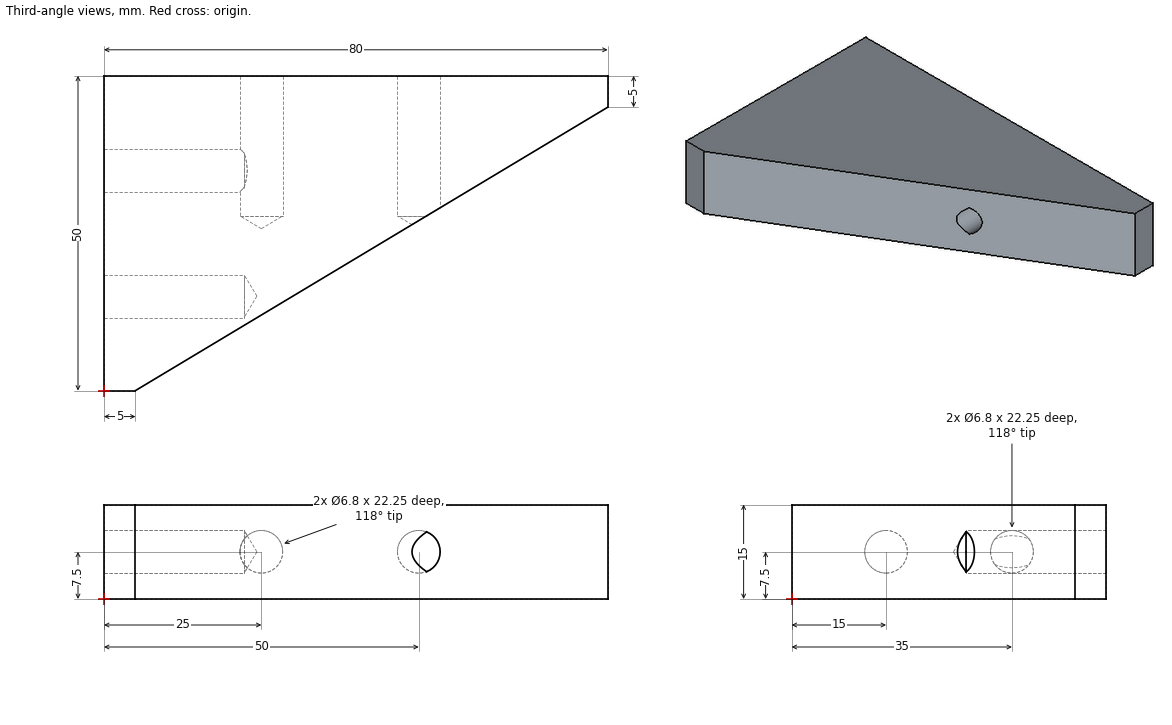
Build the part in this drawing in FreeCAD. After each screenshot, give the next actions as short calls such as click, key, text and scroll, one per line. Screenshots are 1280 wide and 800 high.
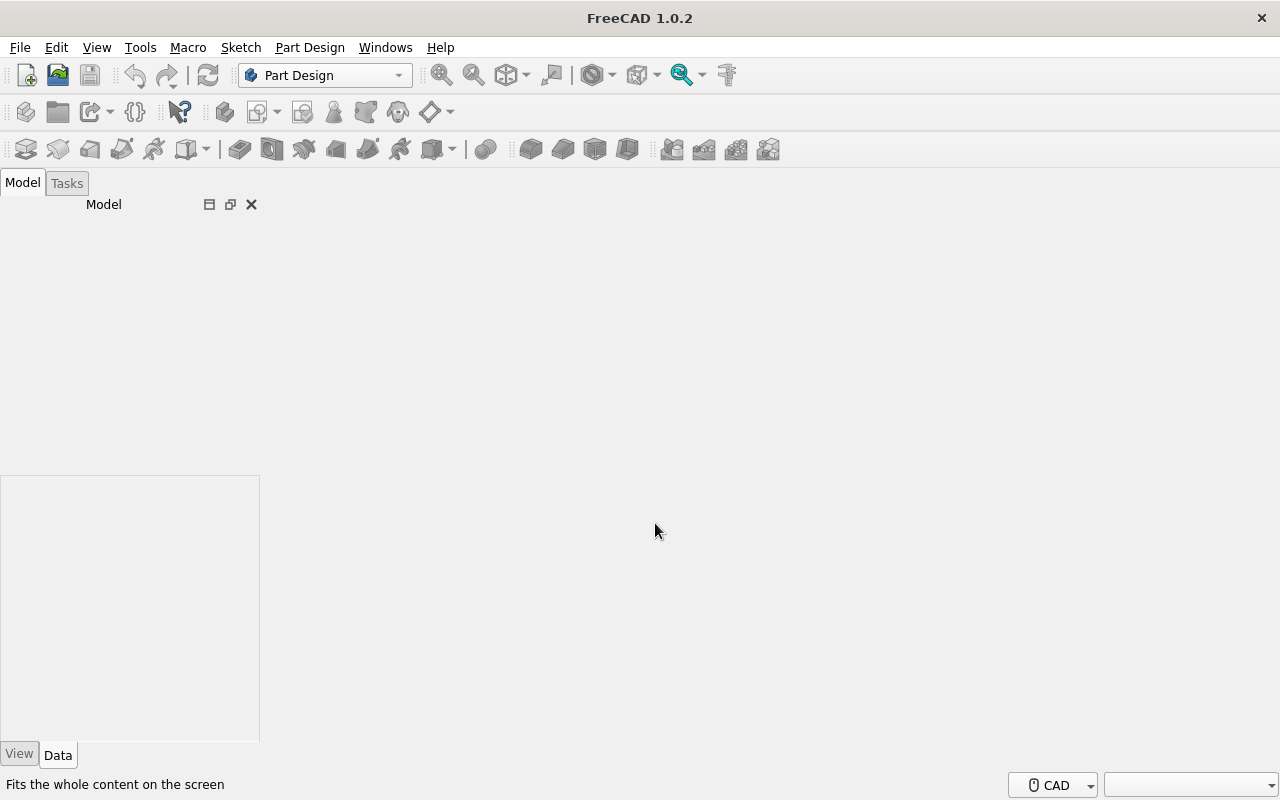
click(26, 76)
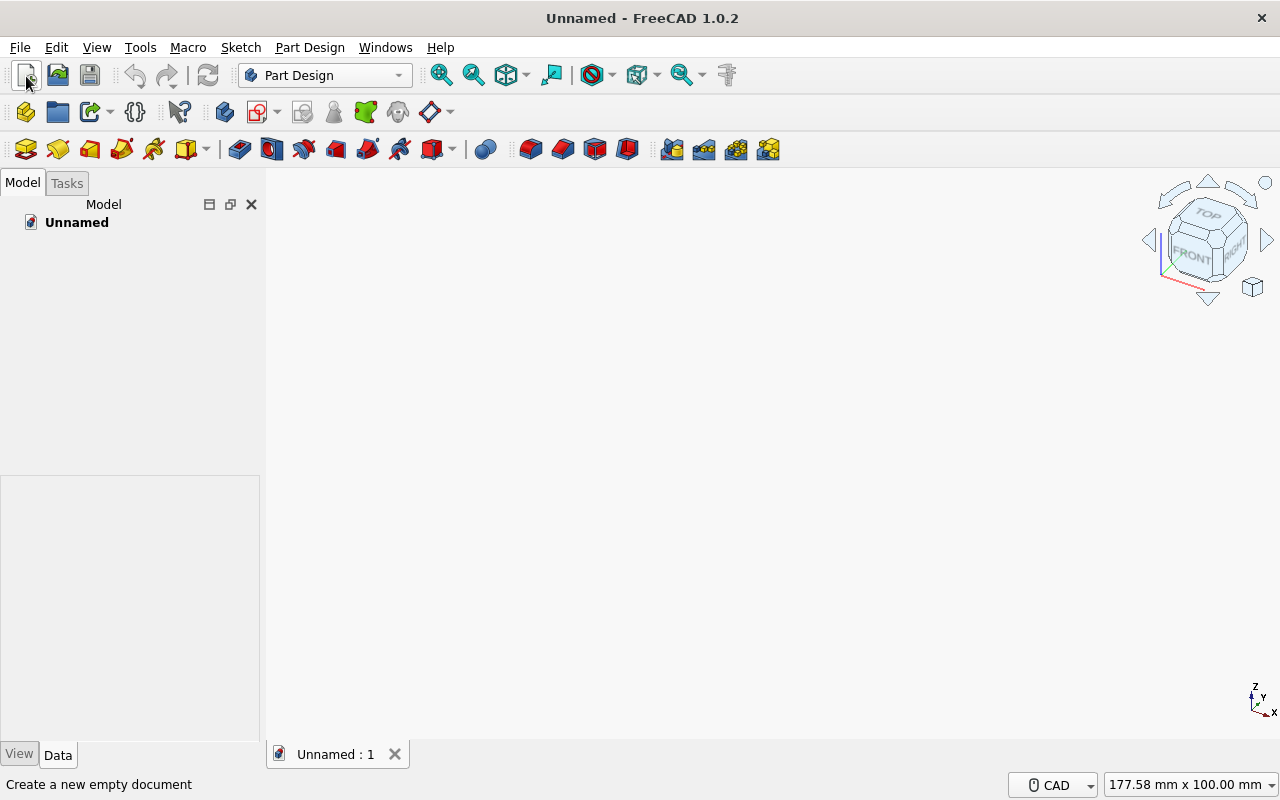
click(258, 112)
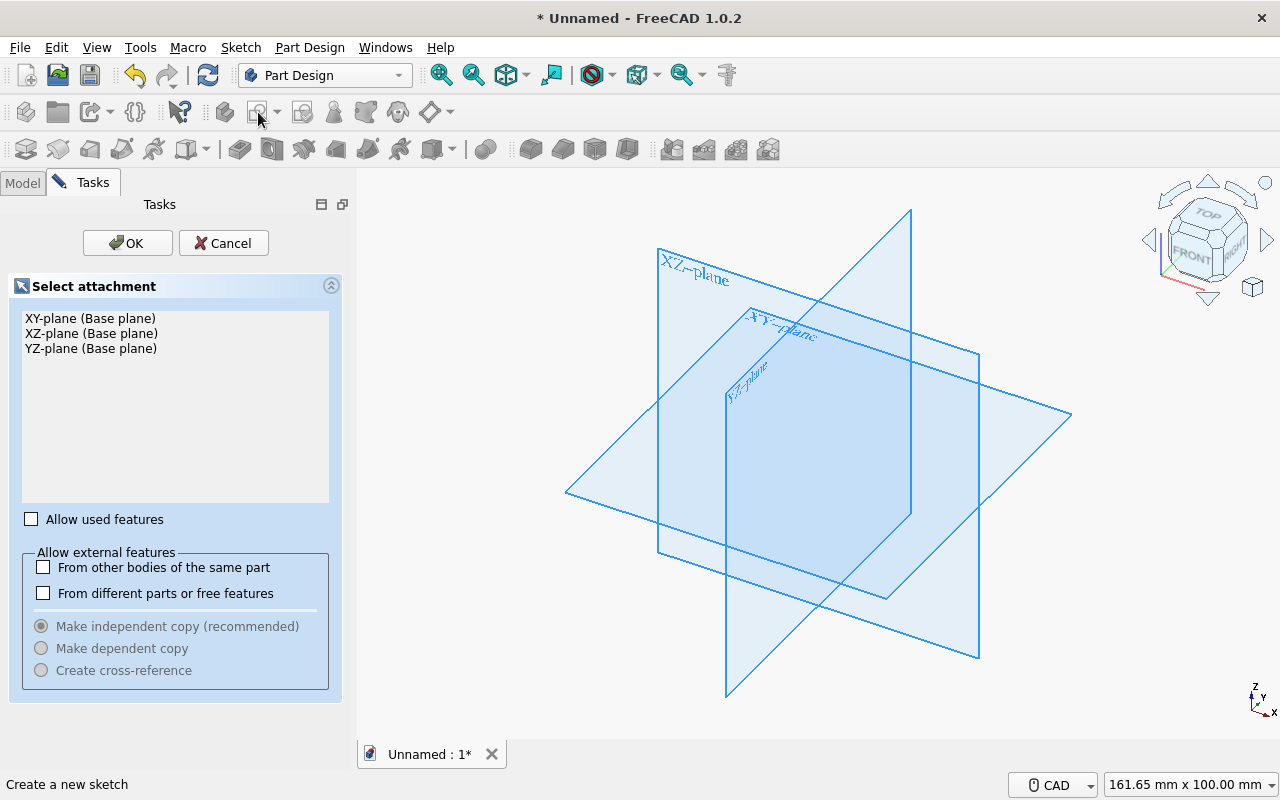
click(82, 318)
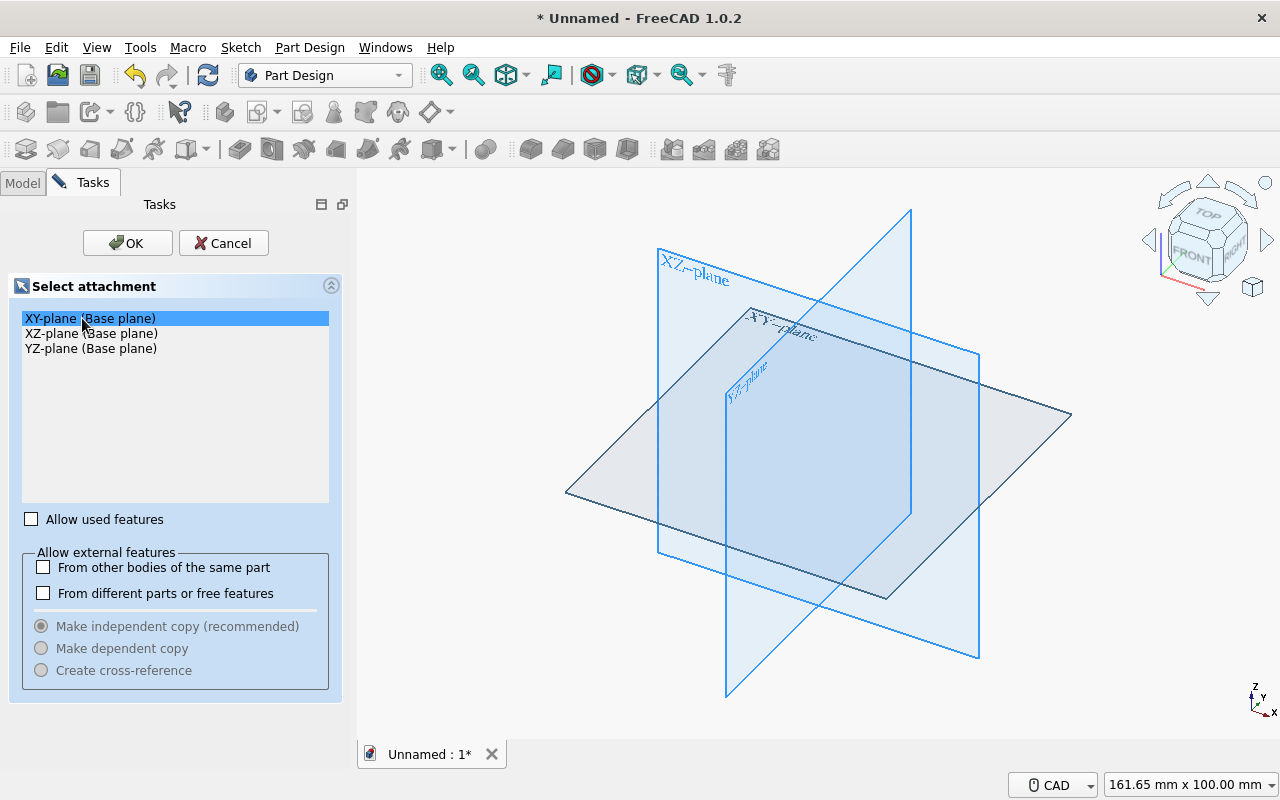
click(128, 243)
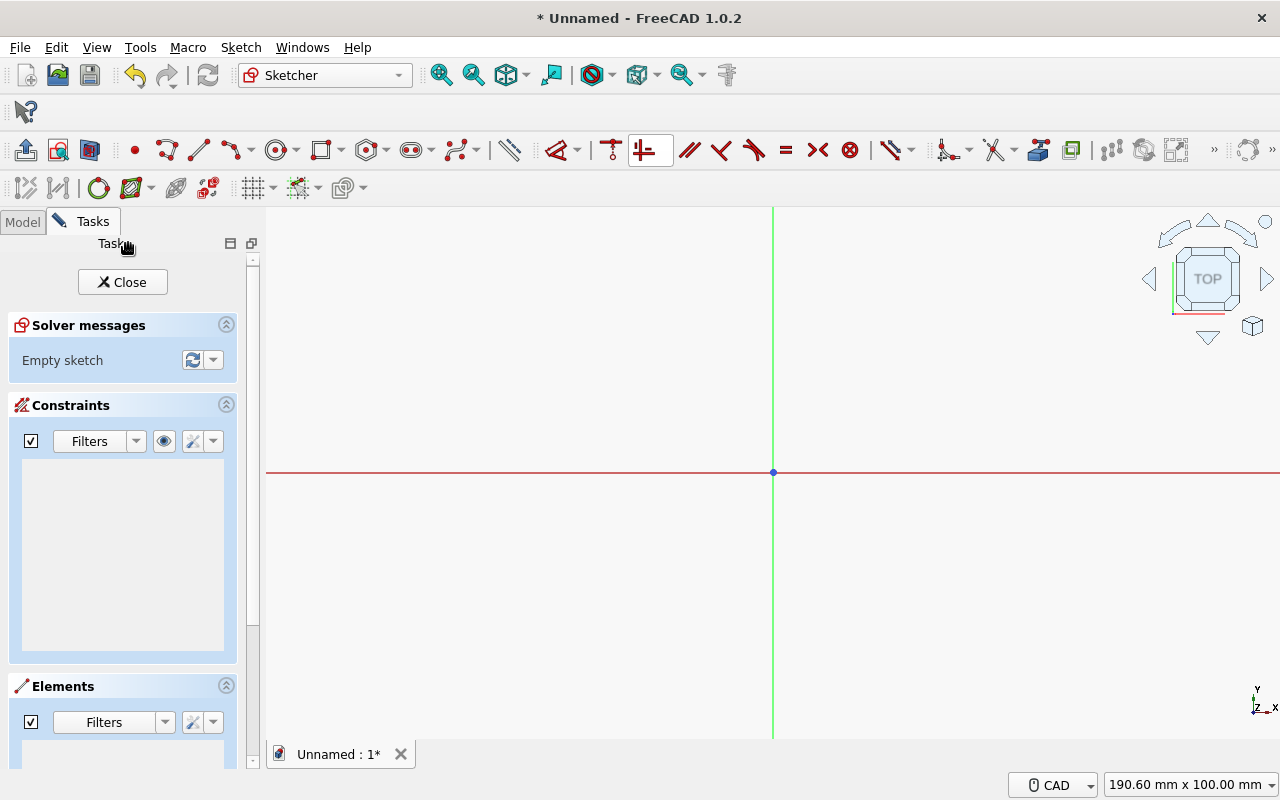
scroll(294, 711, down, 1)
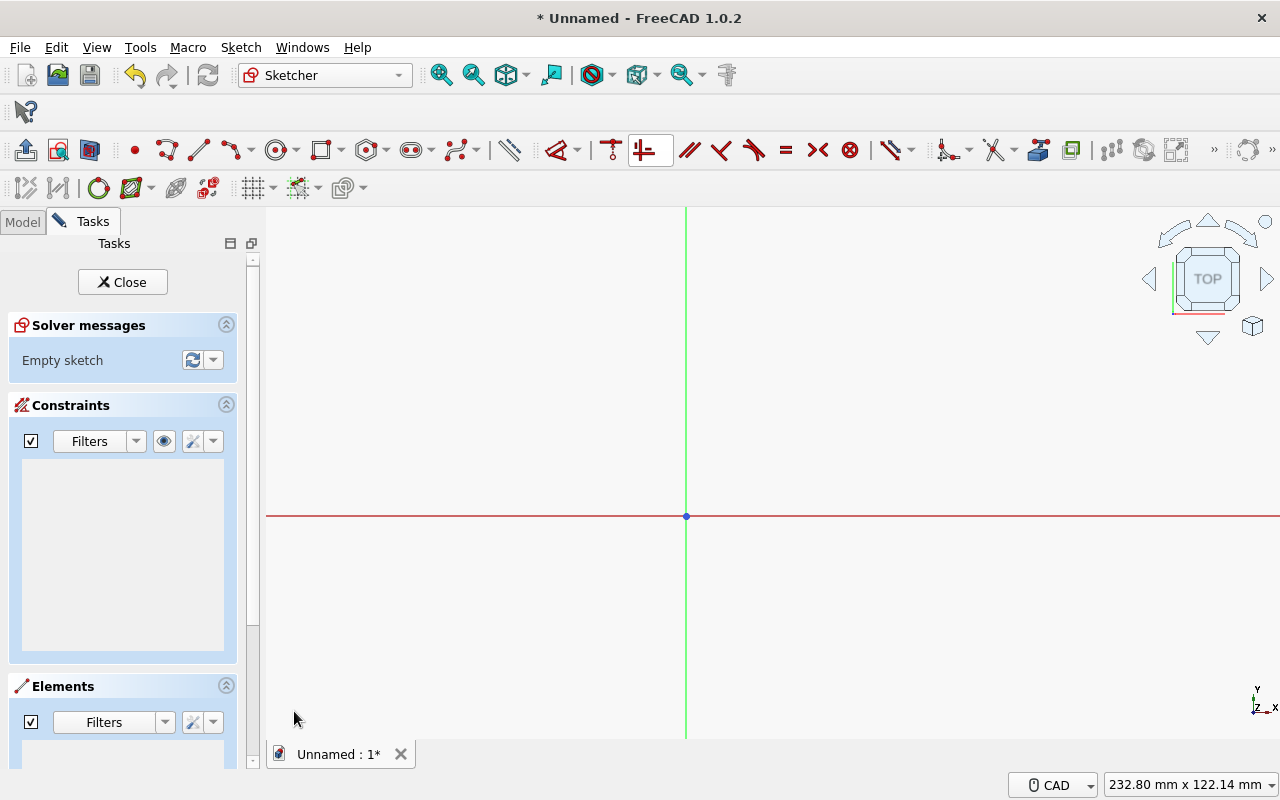
scroll(1115, 274, up, 2)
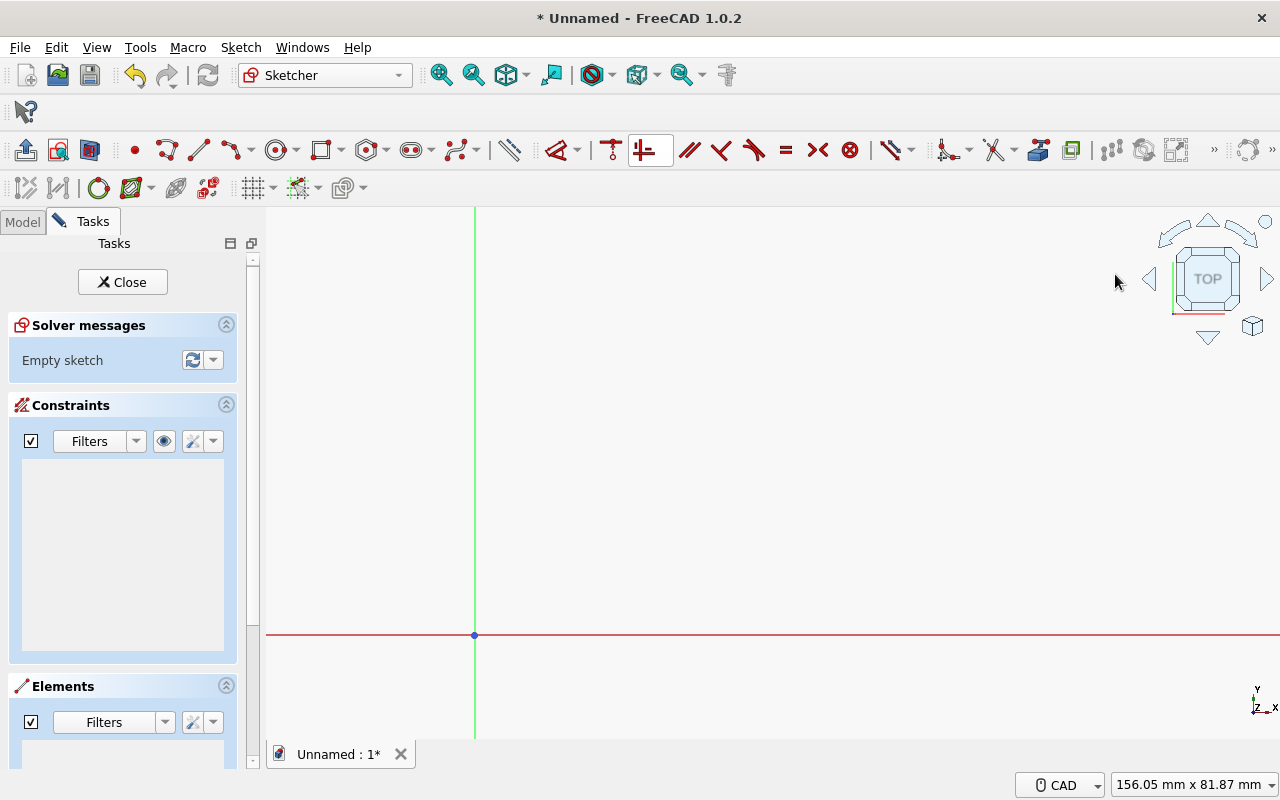
click(168, 150)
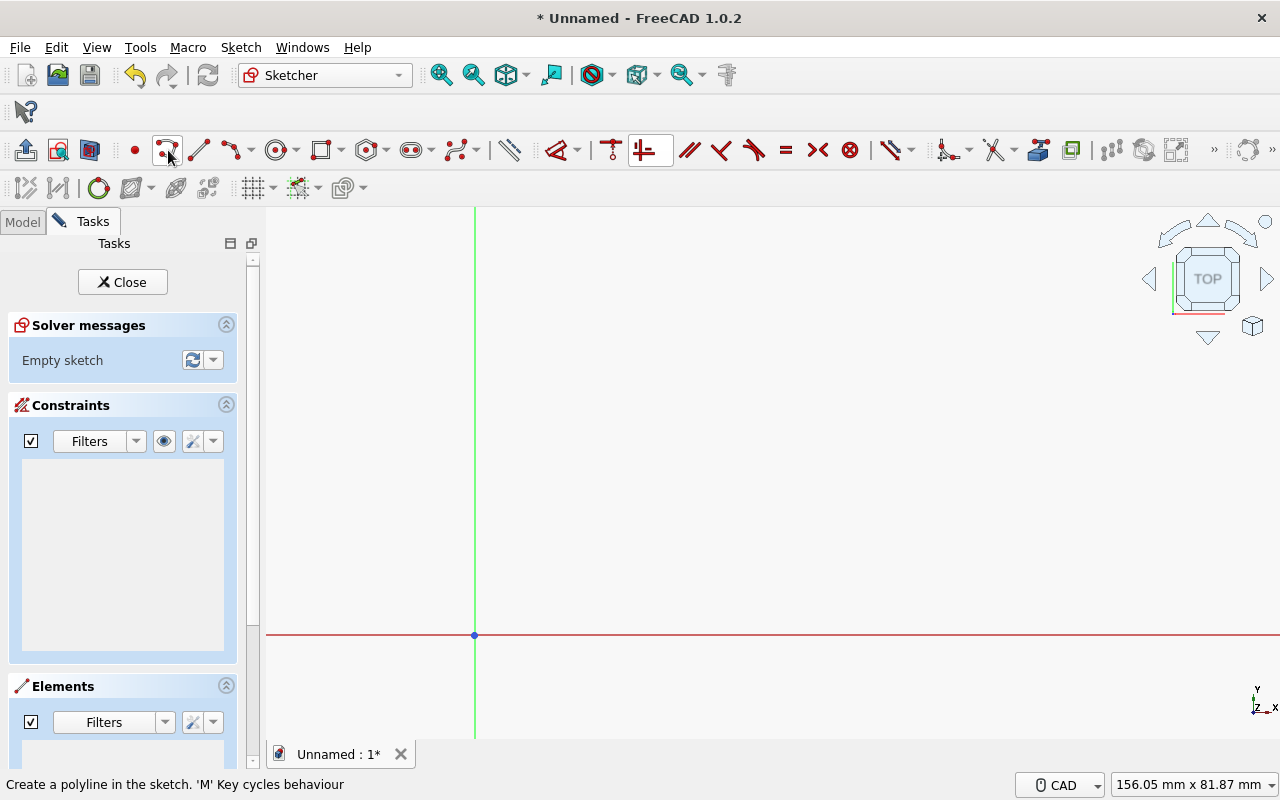
click(475, 635)
click(507, 626)
click(995, 343)
click(995, 311)
click(484, 311)
click(475, 635)
key(Escape)
key(Escape)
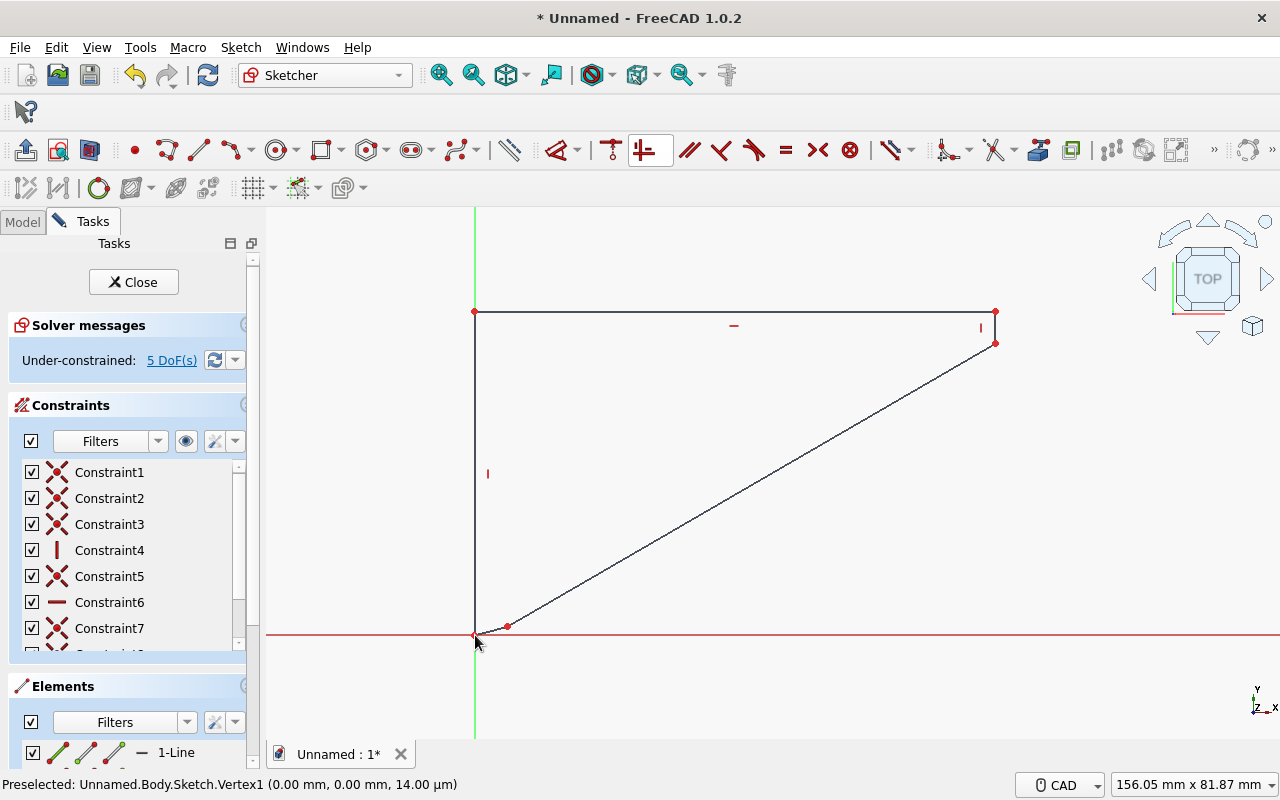
scroll(485, 633, up, 2)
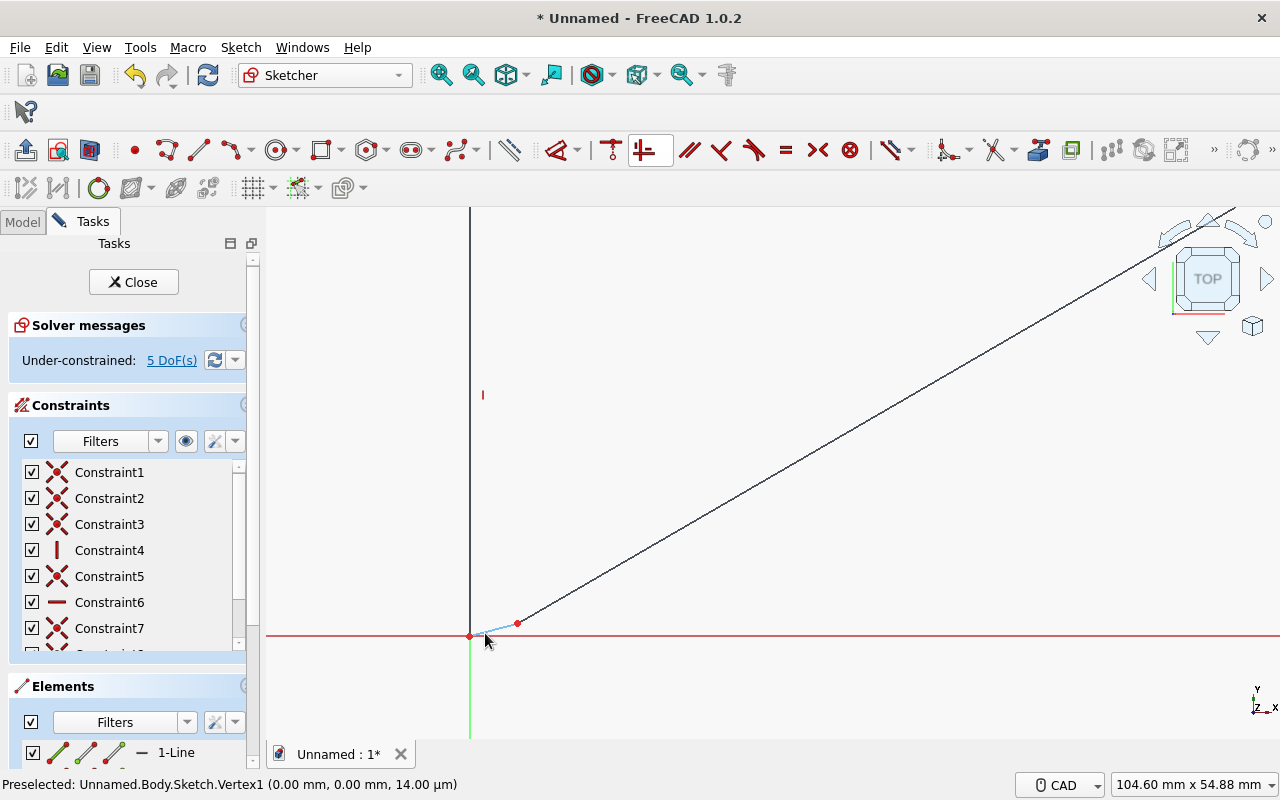
click(484, 632)